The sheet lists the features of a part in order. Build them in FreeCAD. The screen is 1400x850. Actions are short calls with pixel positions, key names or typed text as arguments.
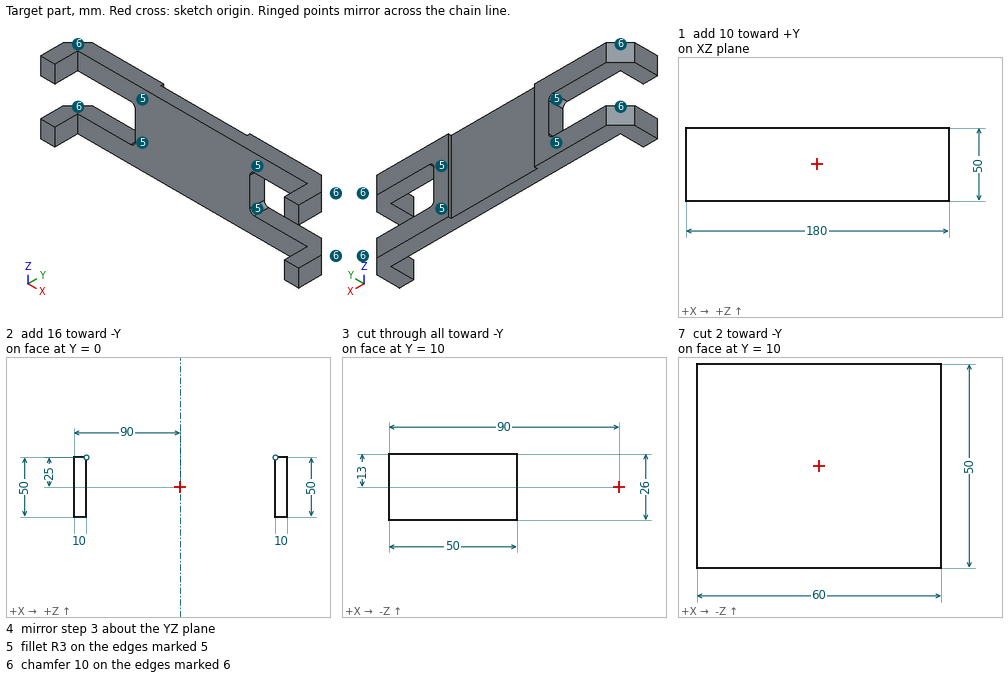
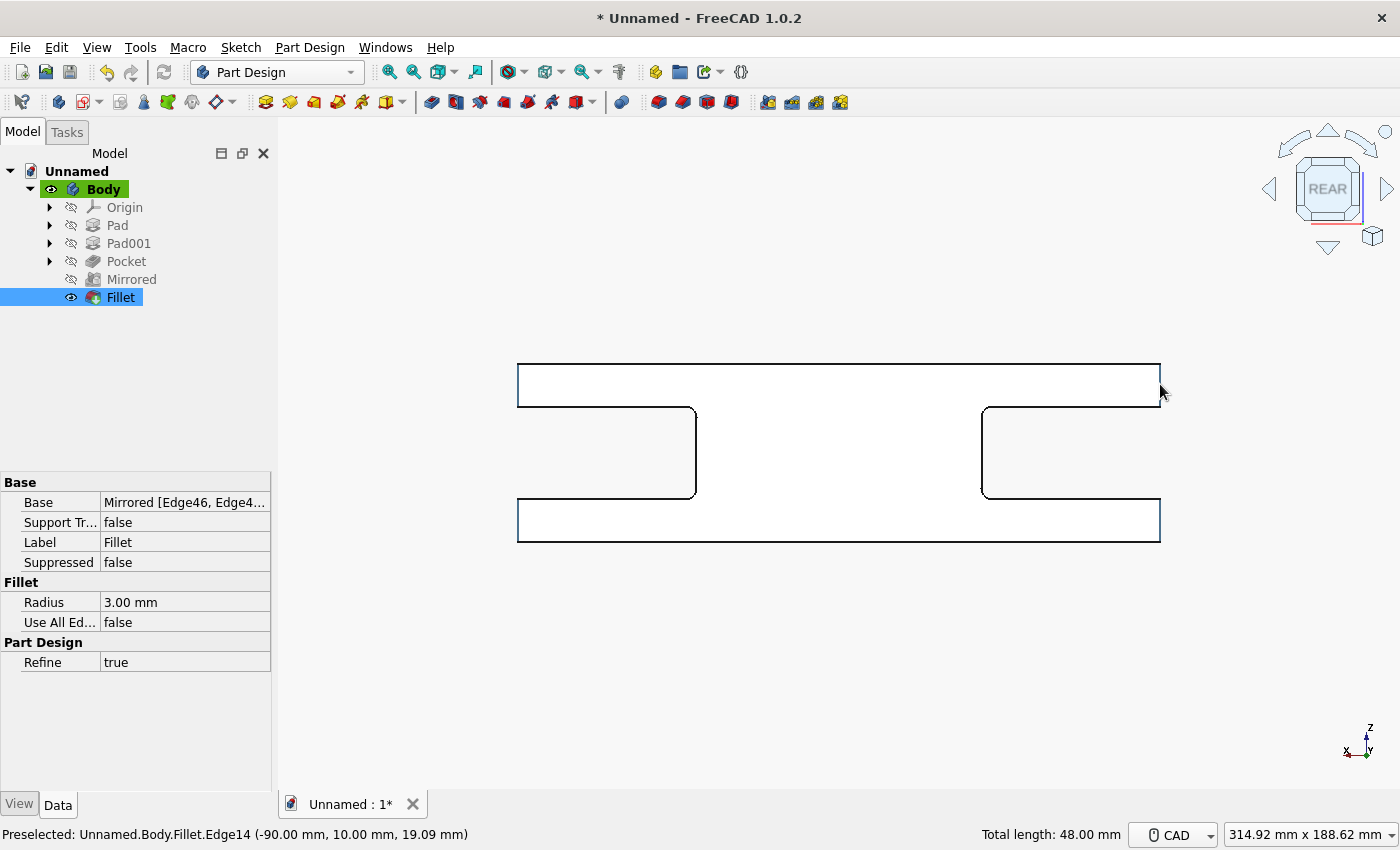
click(684, 102)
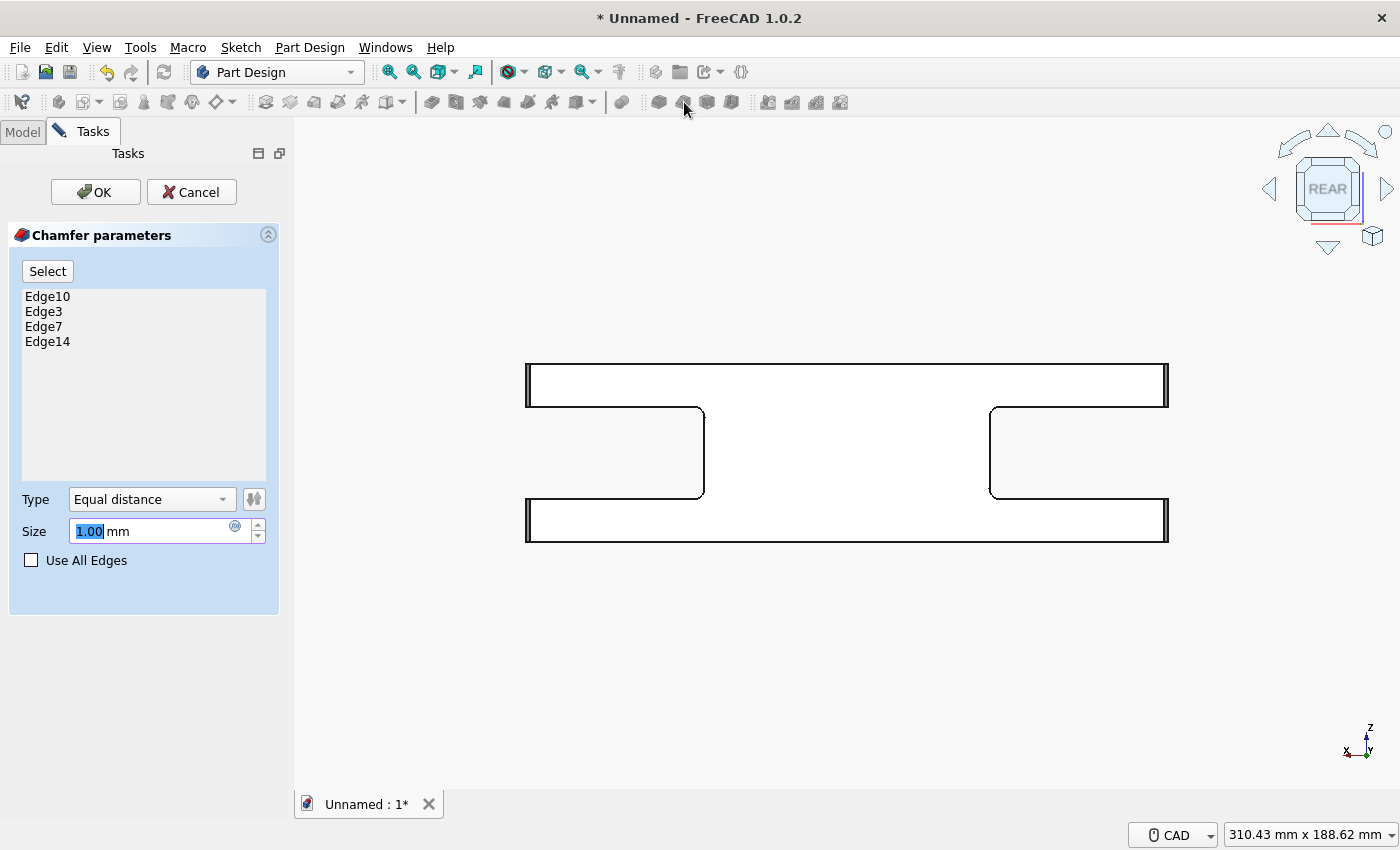
text(10)
key(Tab)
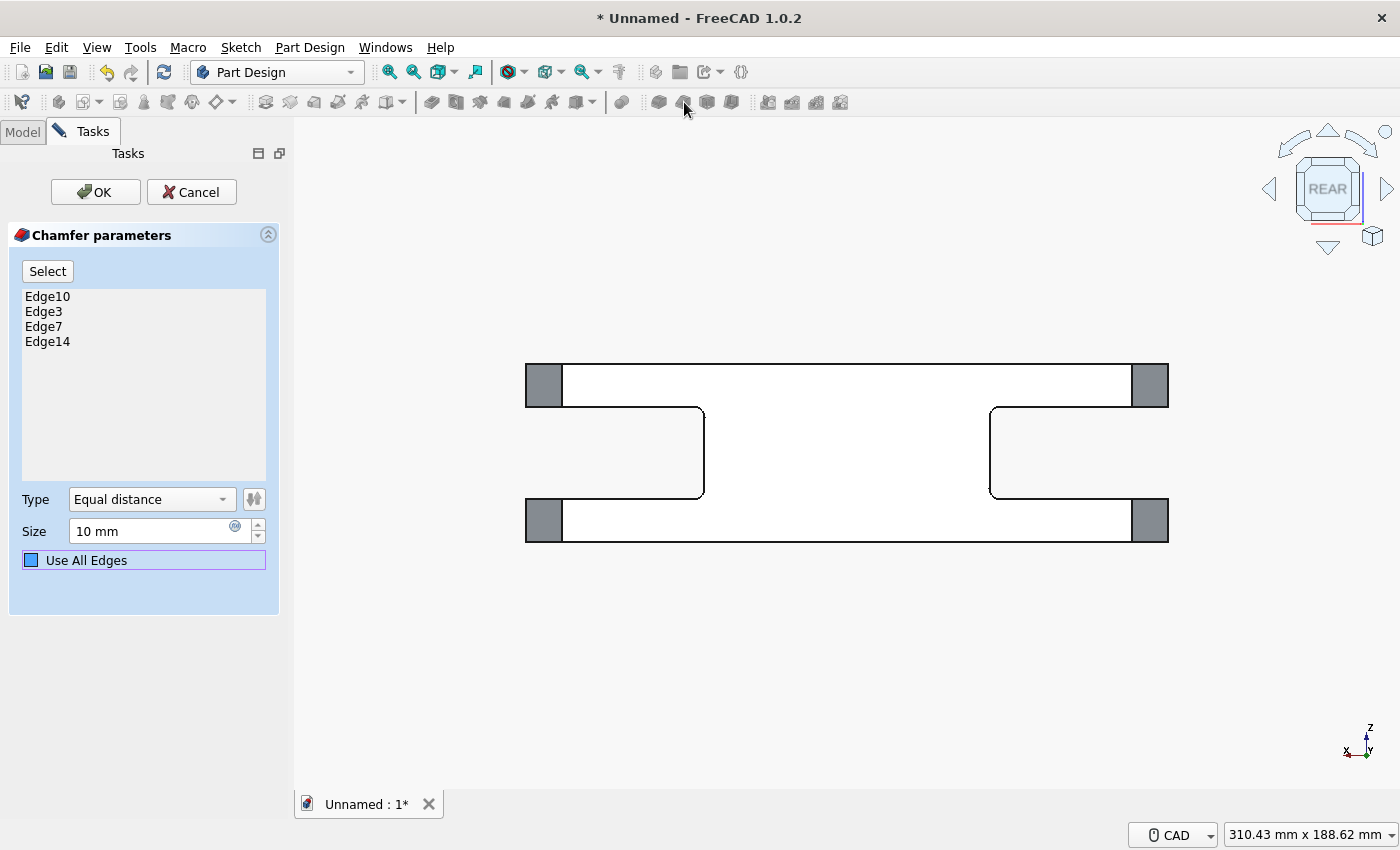
click(96, 192)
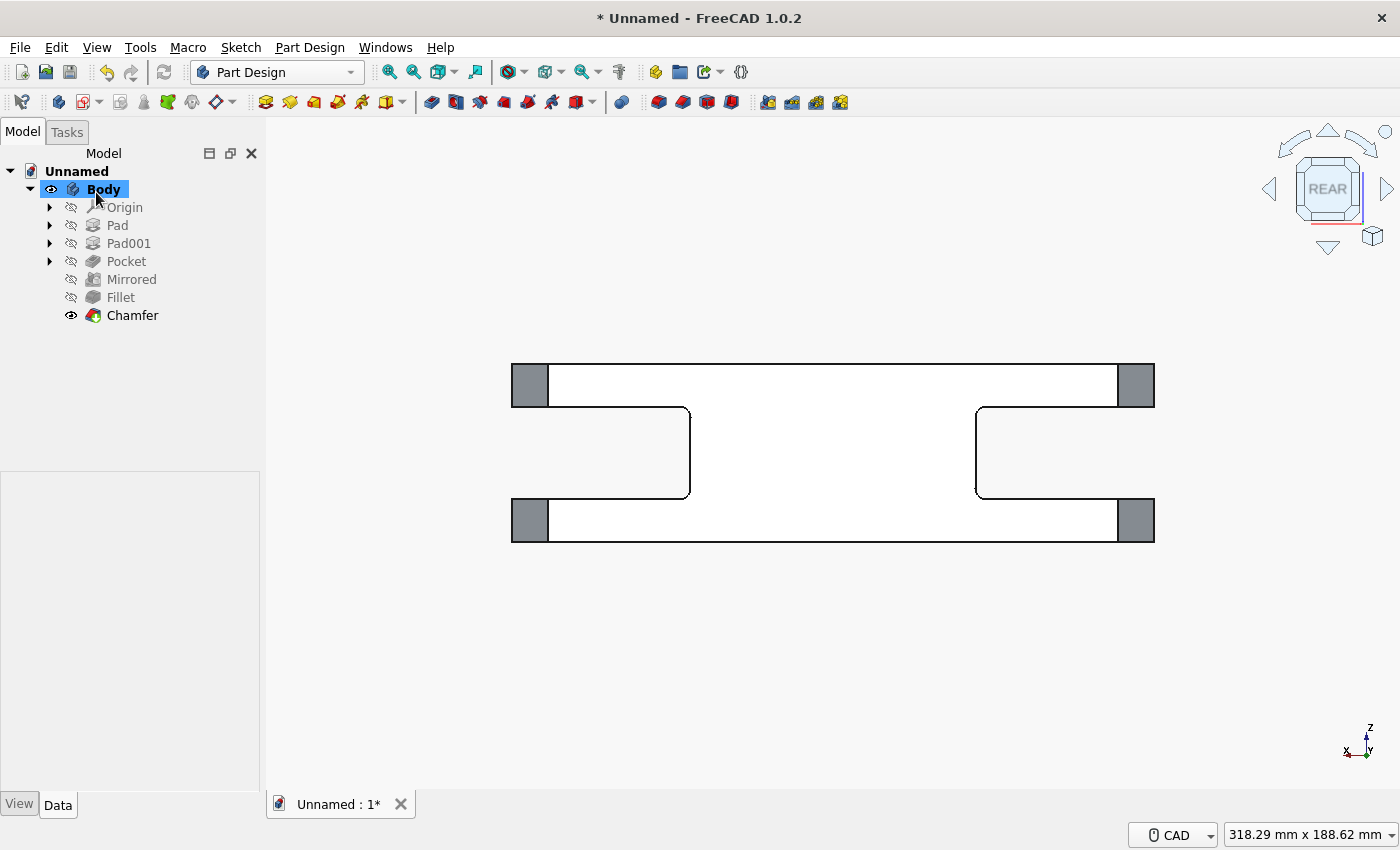
click(833, 452)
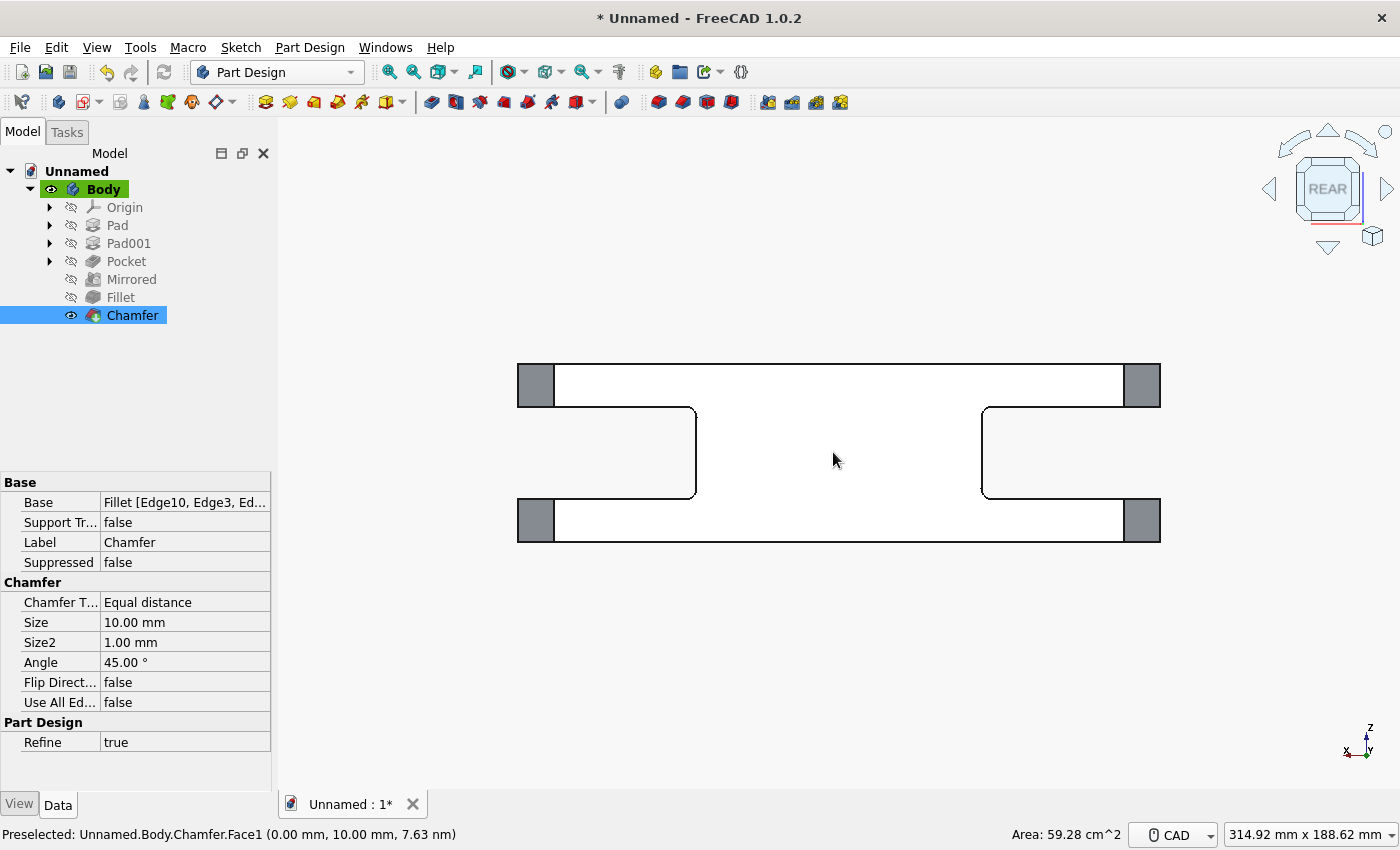
click(84, 102)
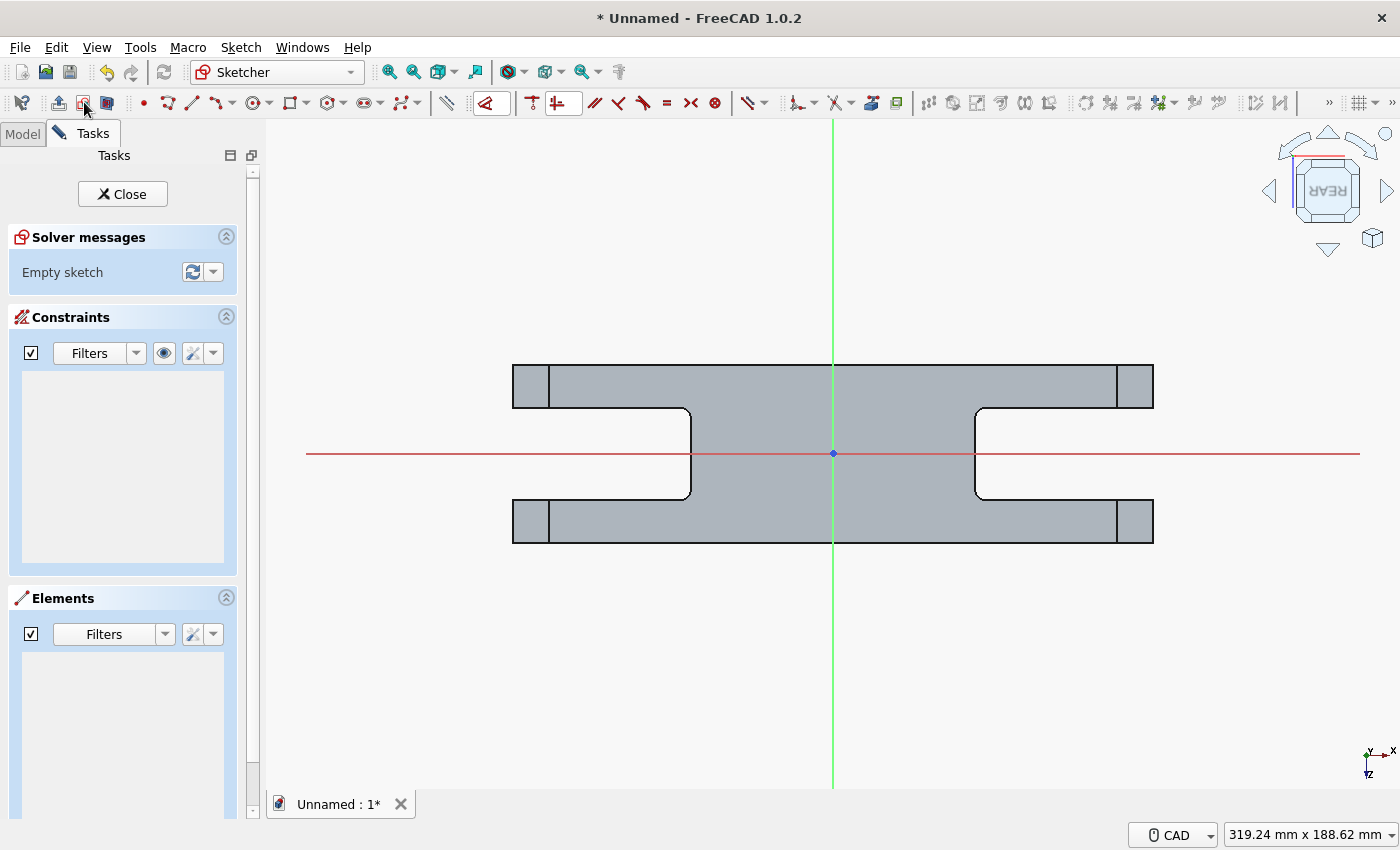
scroll(889, 454, up, 4)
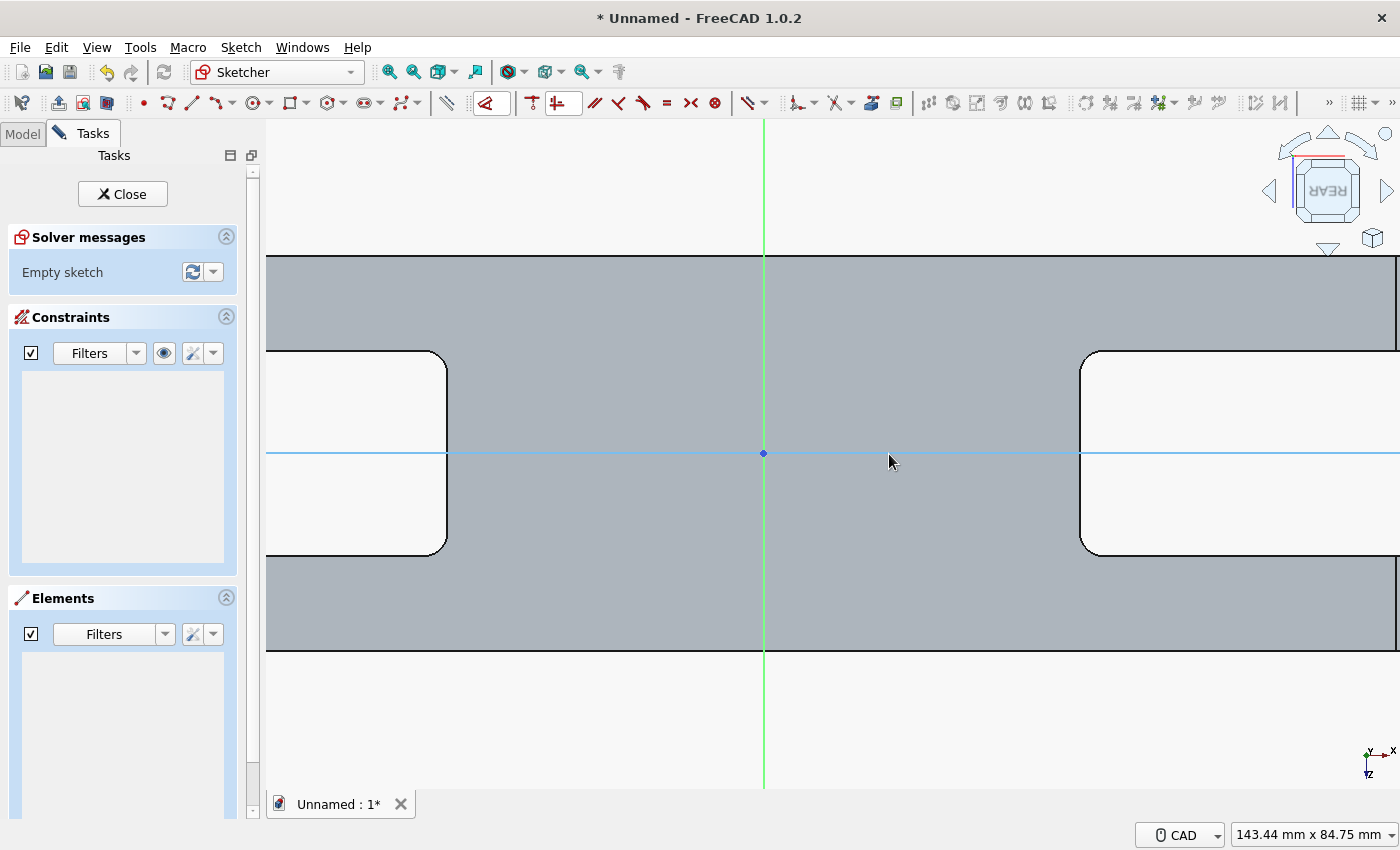
key(g)
key(v)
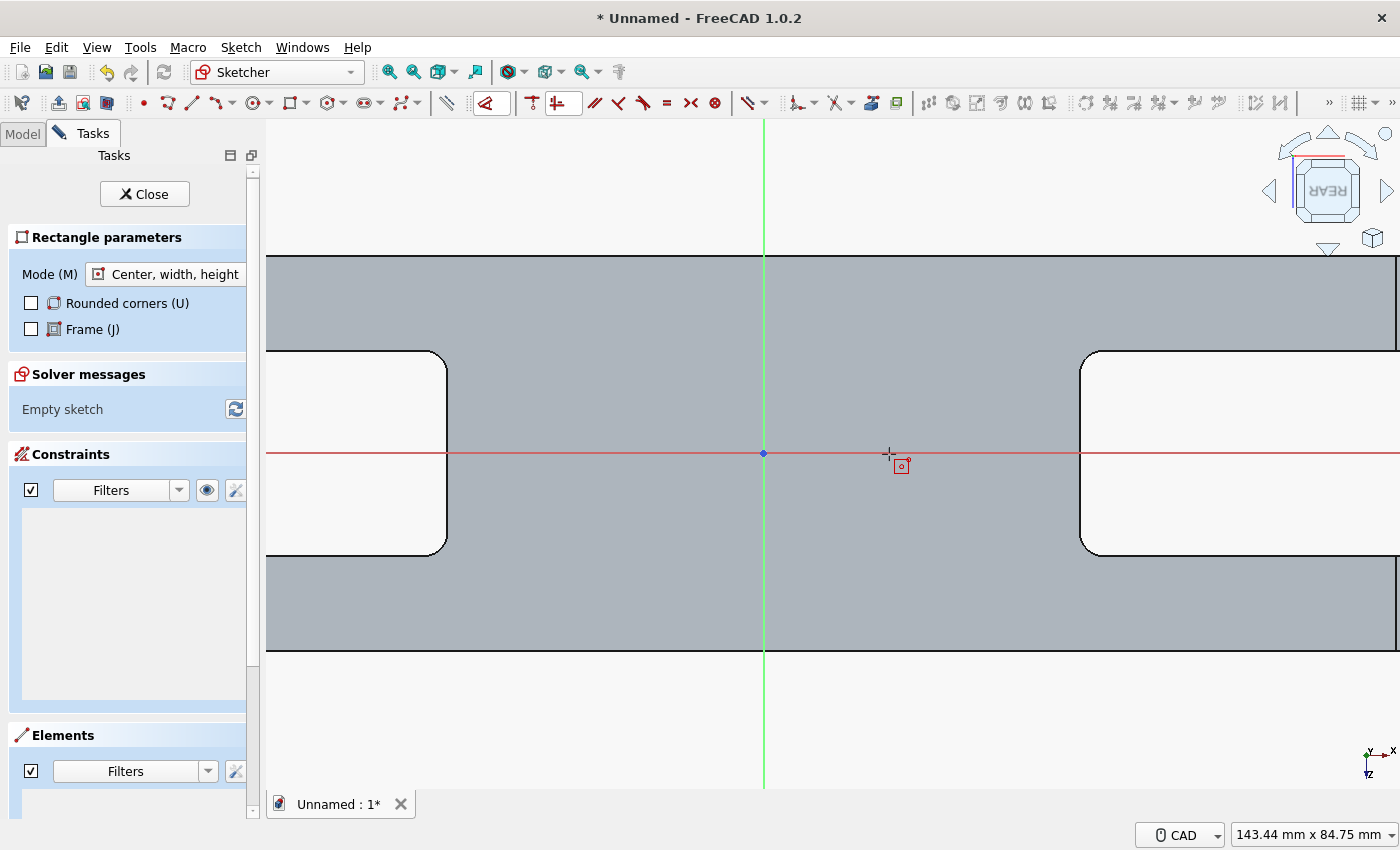
click(764, 453)
move(1001, 256)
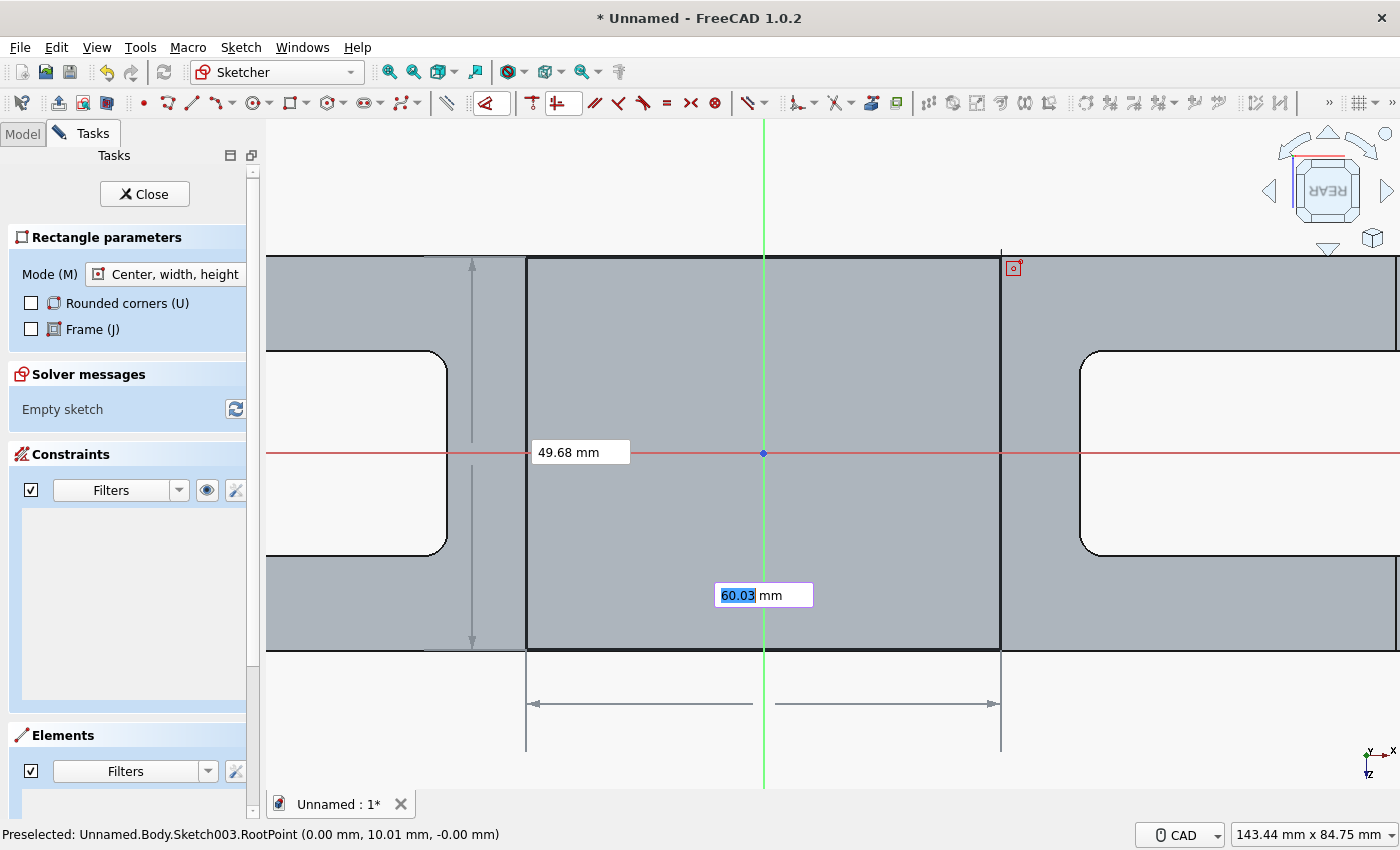
text(60)
key(Tab)
text(50)
key(Return)
key(Escape)